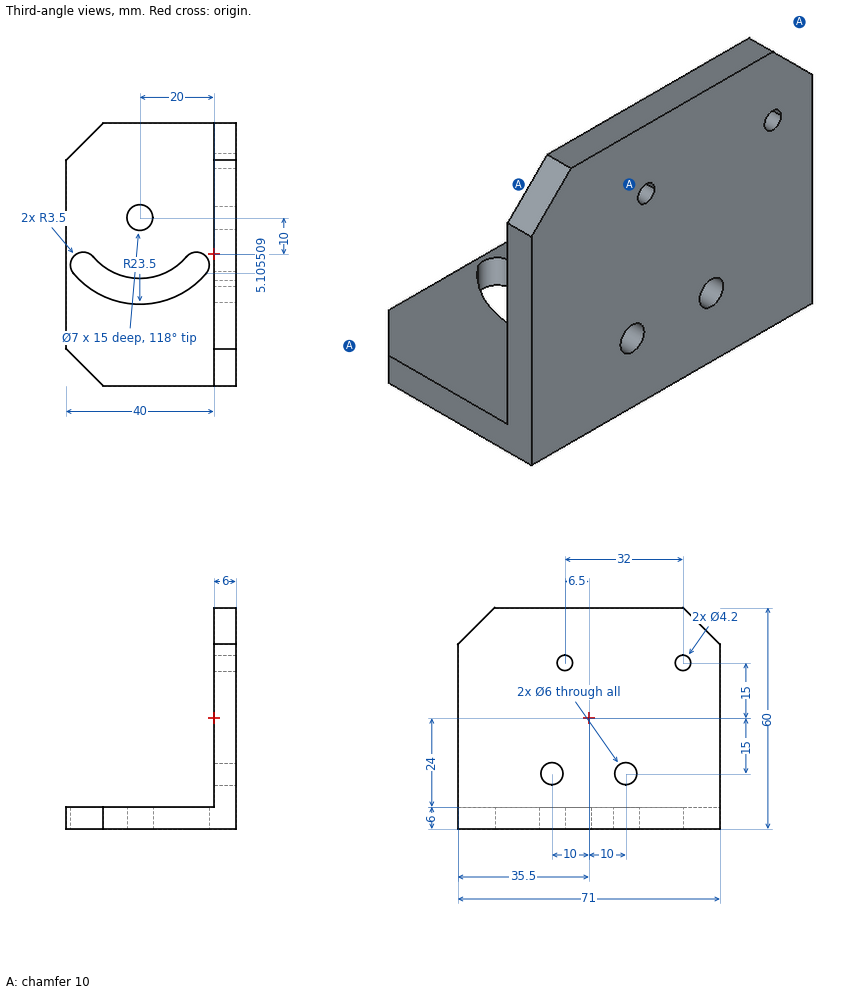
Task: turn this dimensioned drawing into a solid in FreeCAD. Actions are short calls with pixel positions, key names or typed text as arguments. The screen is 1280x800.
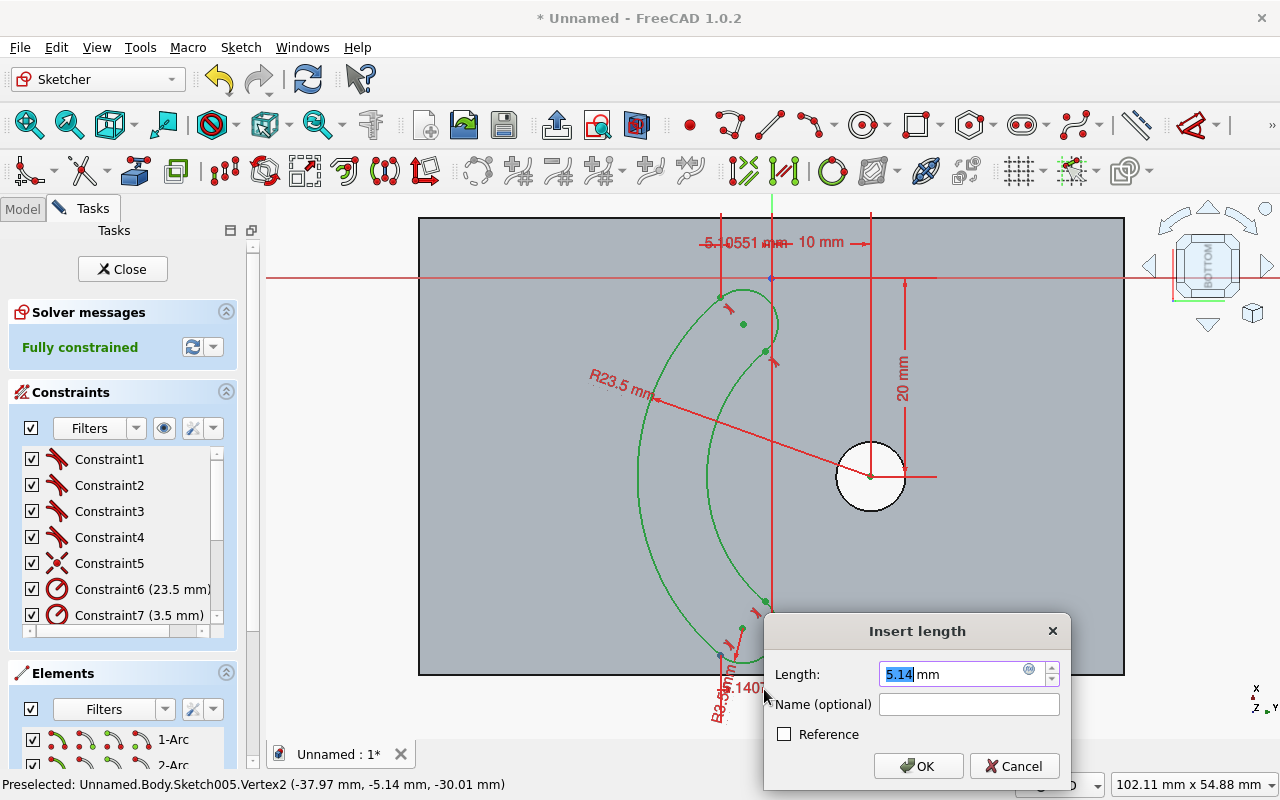
text(5.105509)
key(Return)
key(Escape)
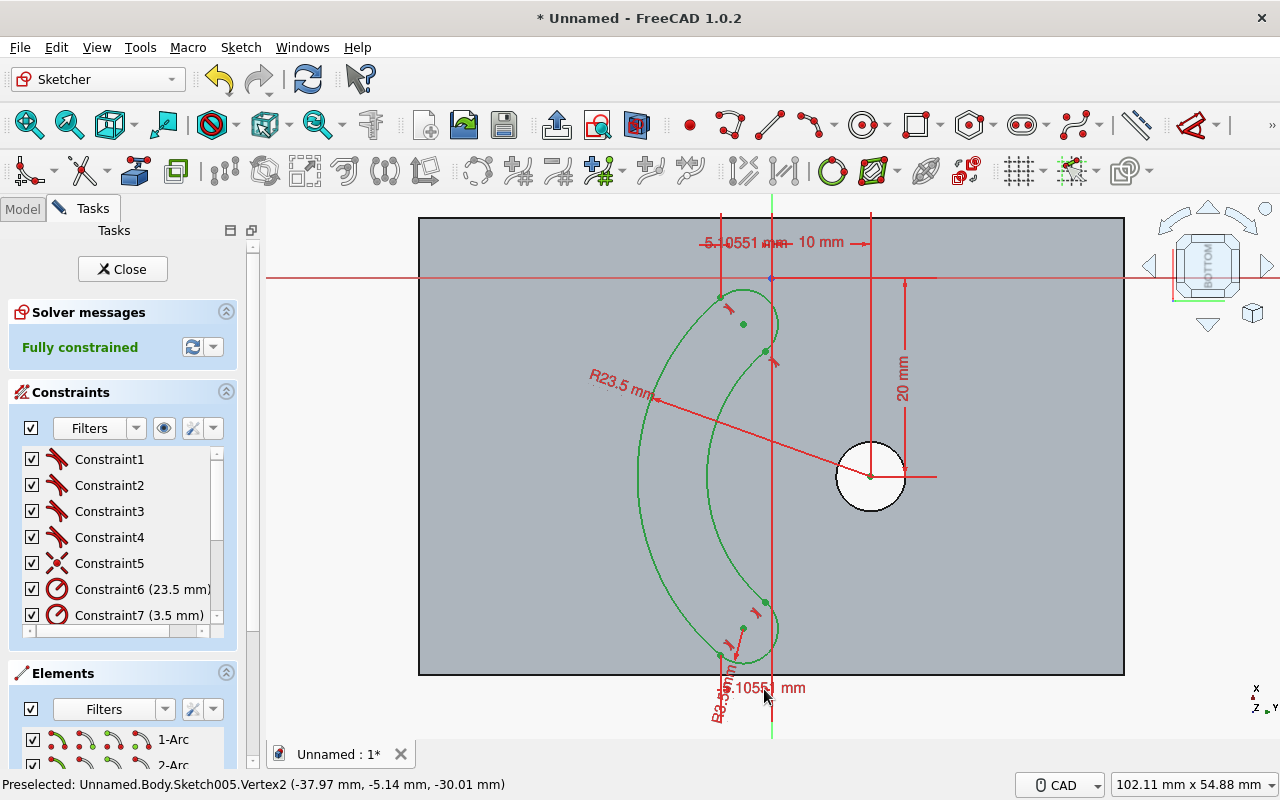
click(123, 269)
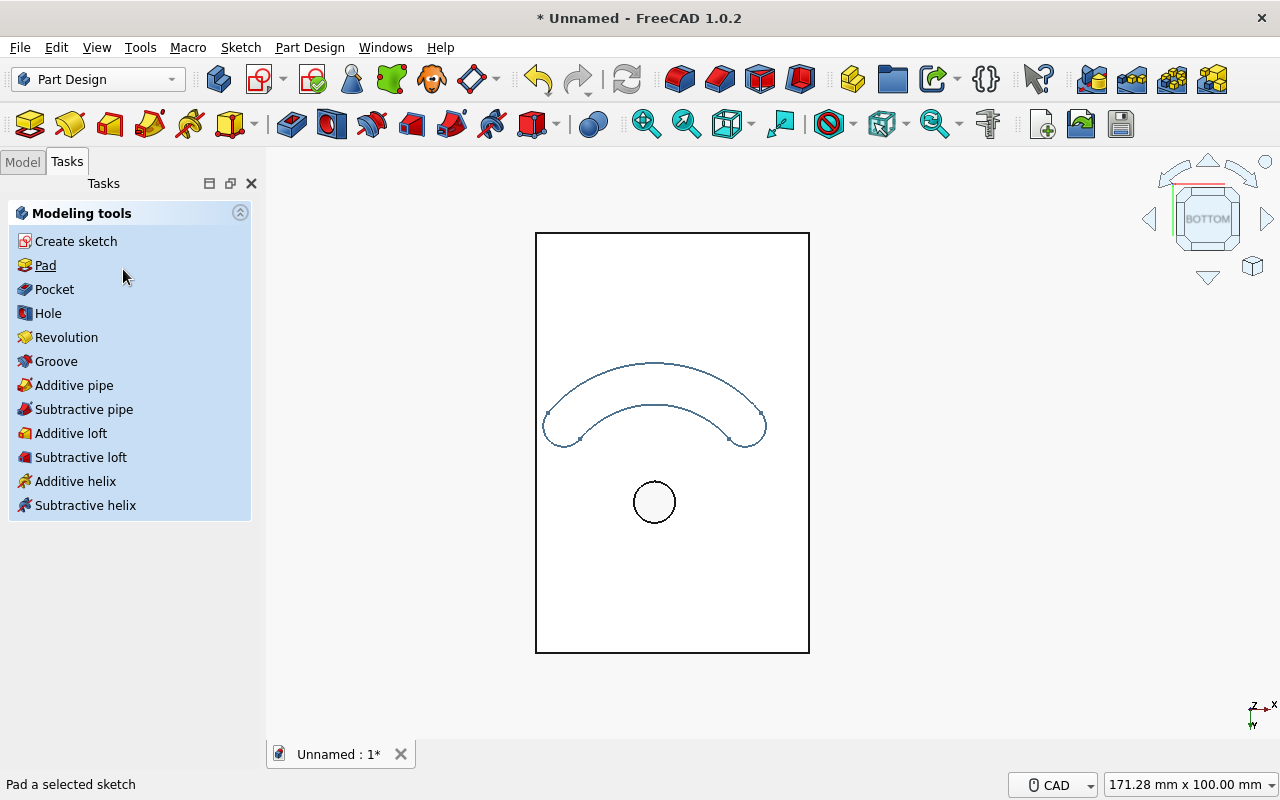
click(292, 124)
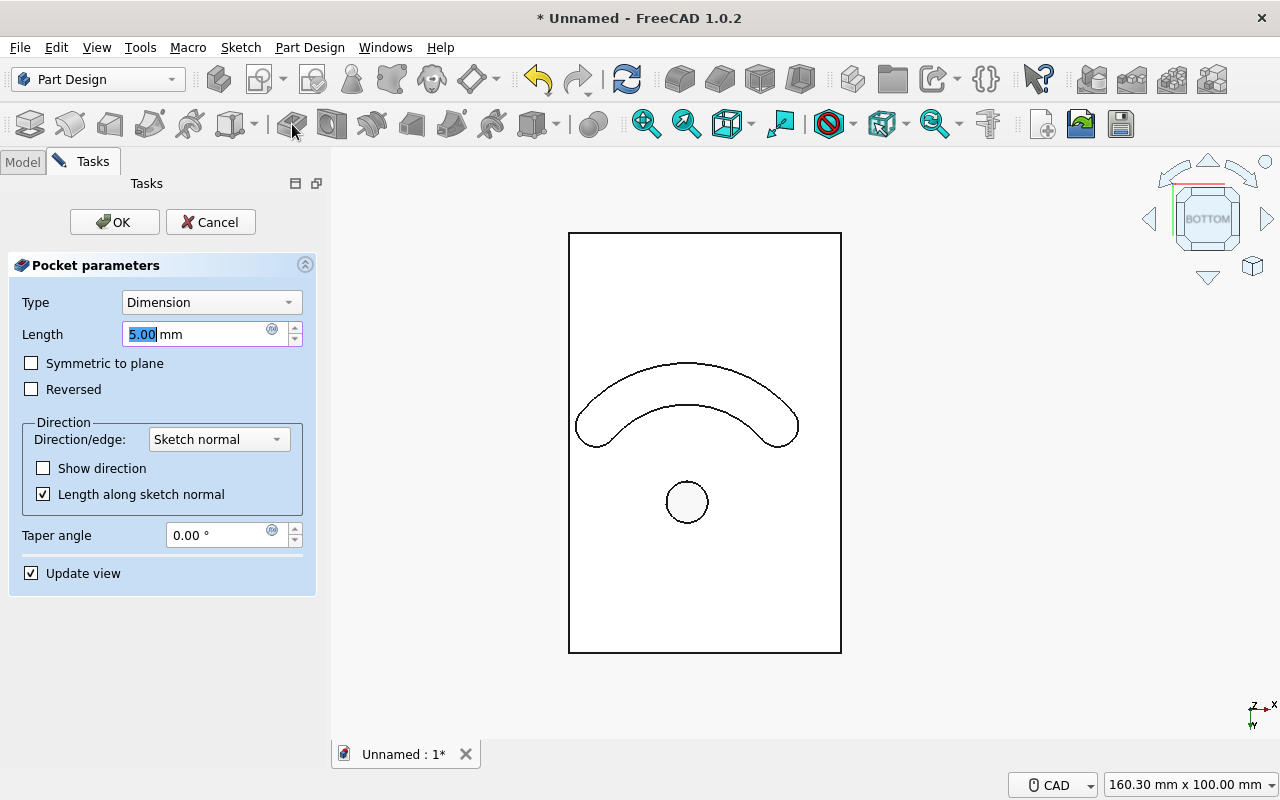
click(212, 302)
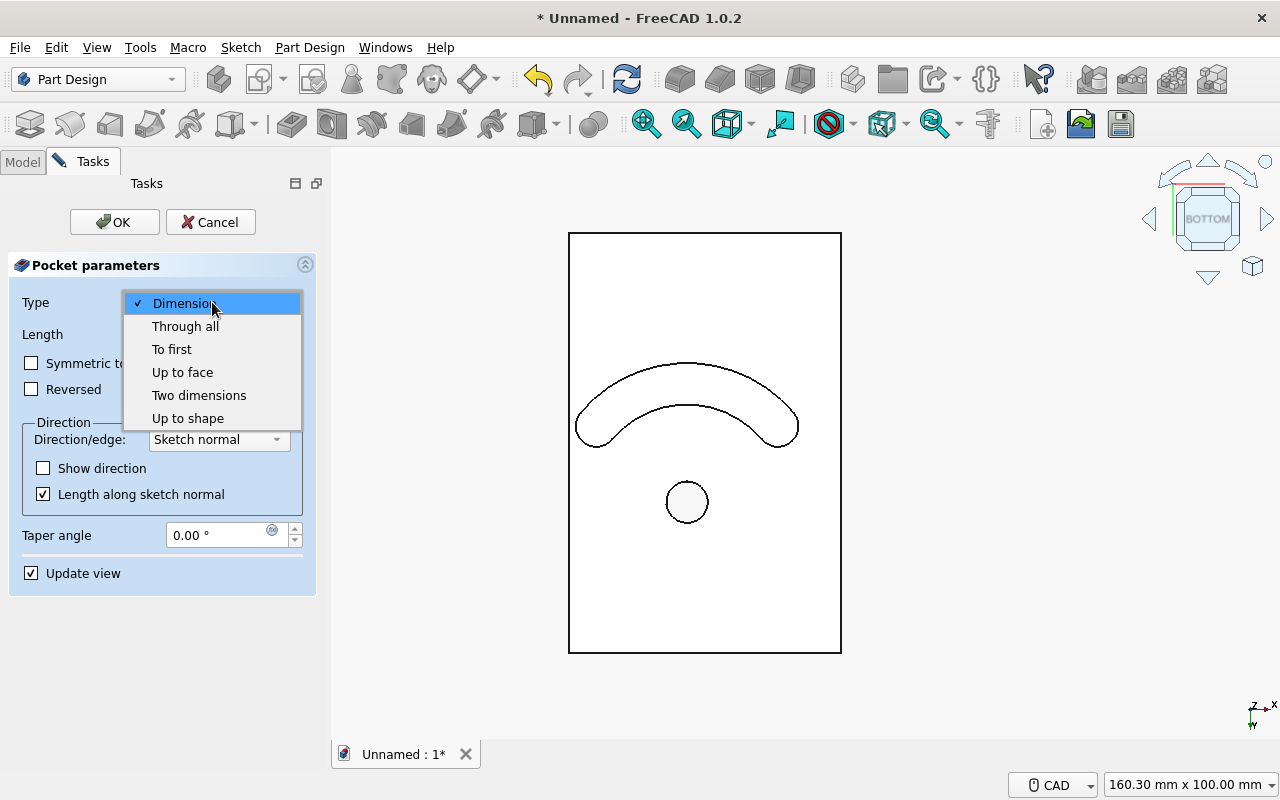
click(212, 326)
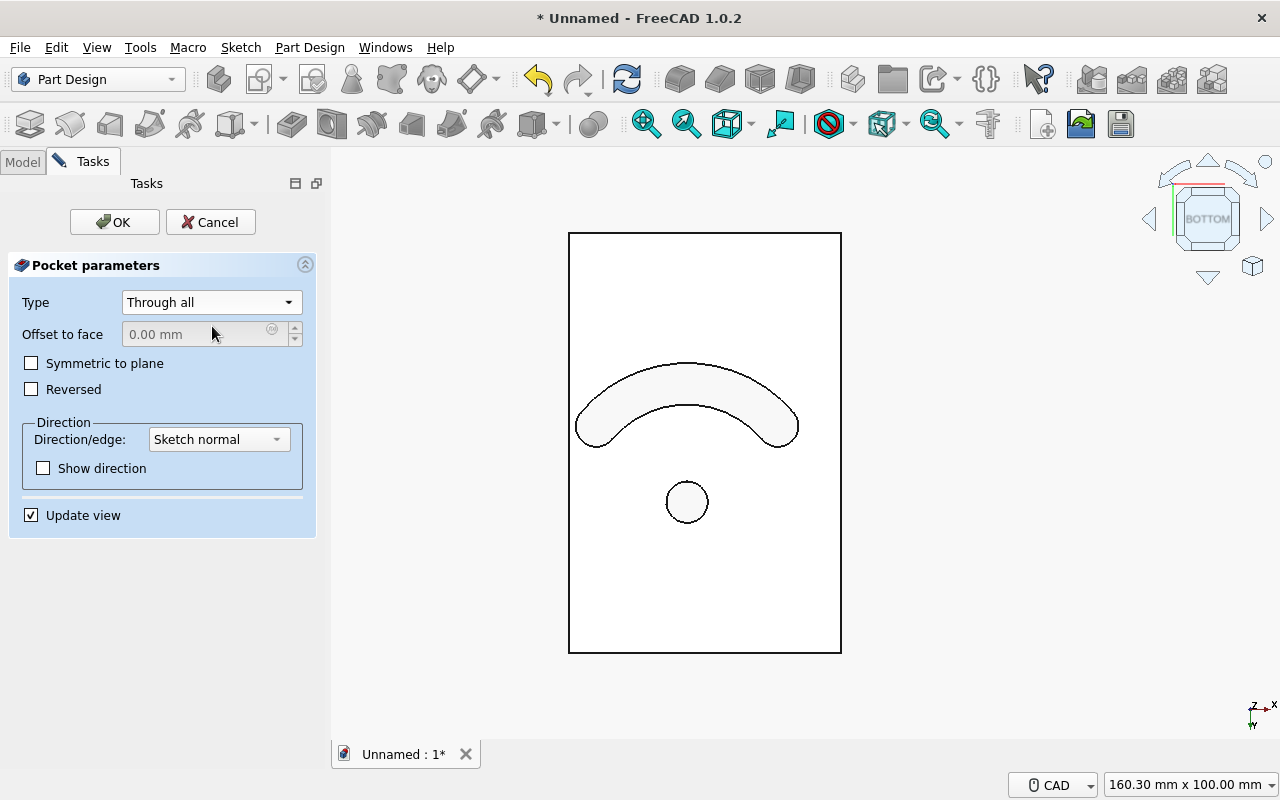
click(115, 222)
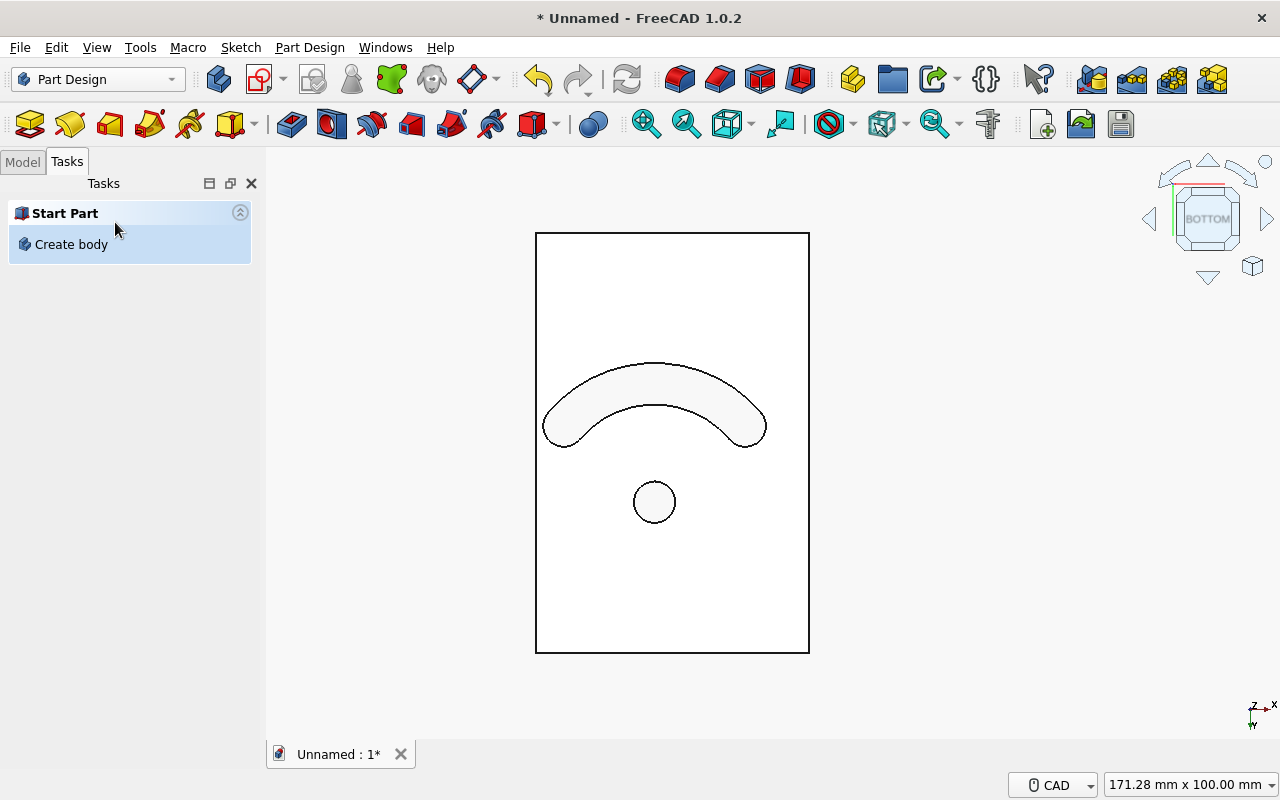
key(0)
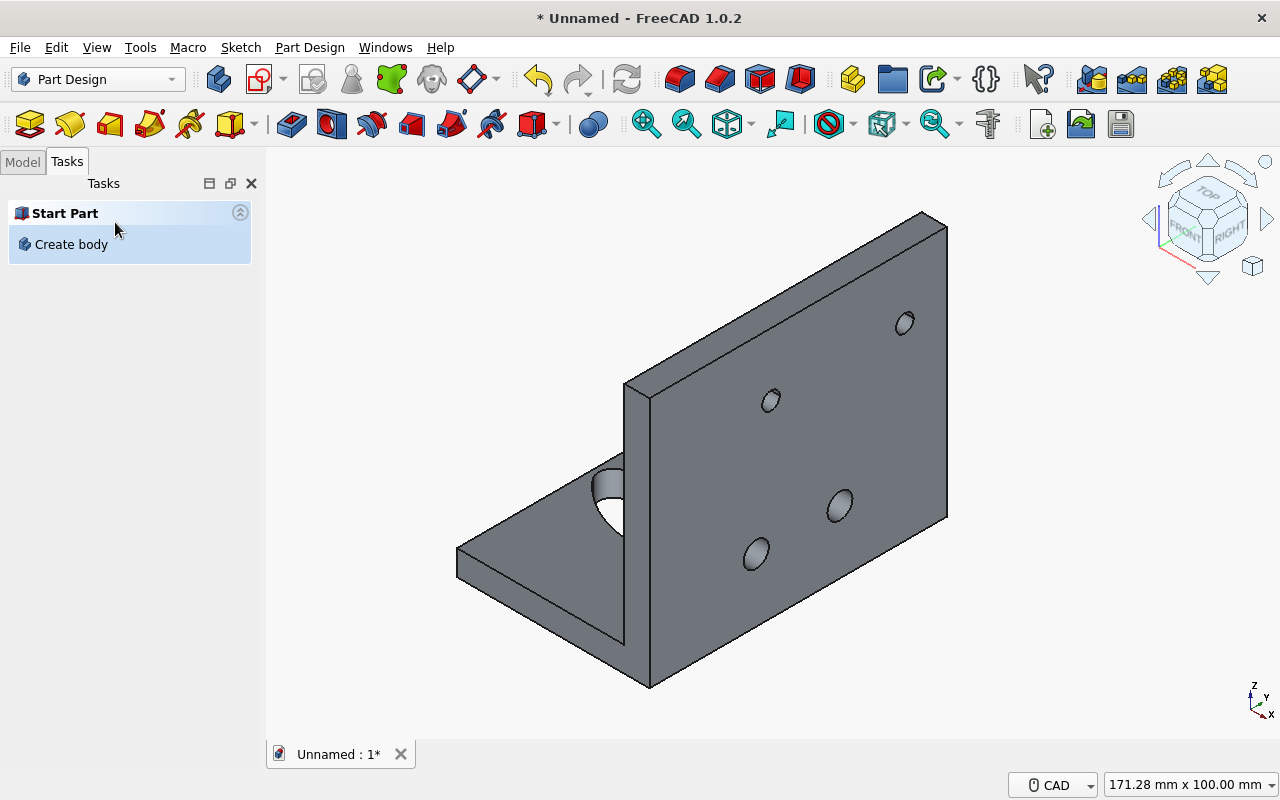
click(648, 124)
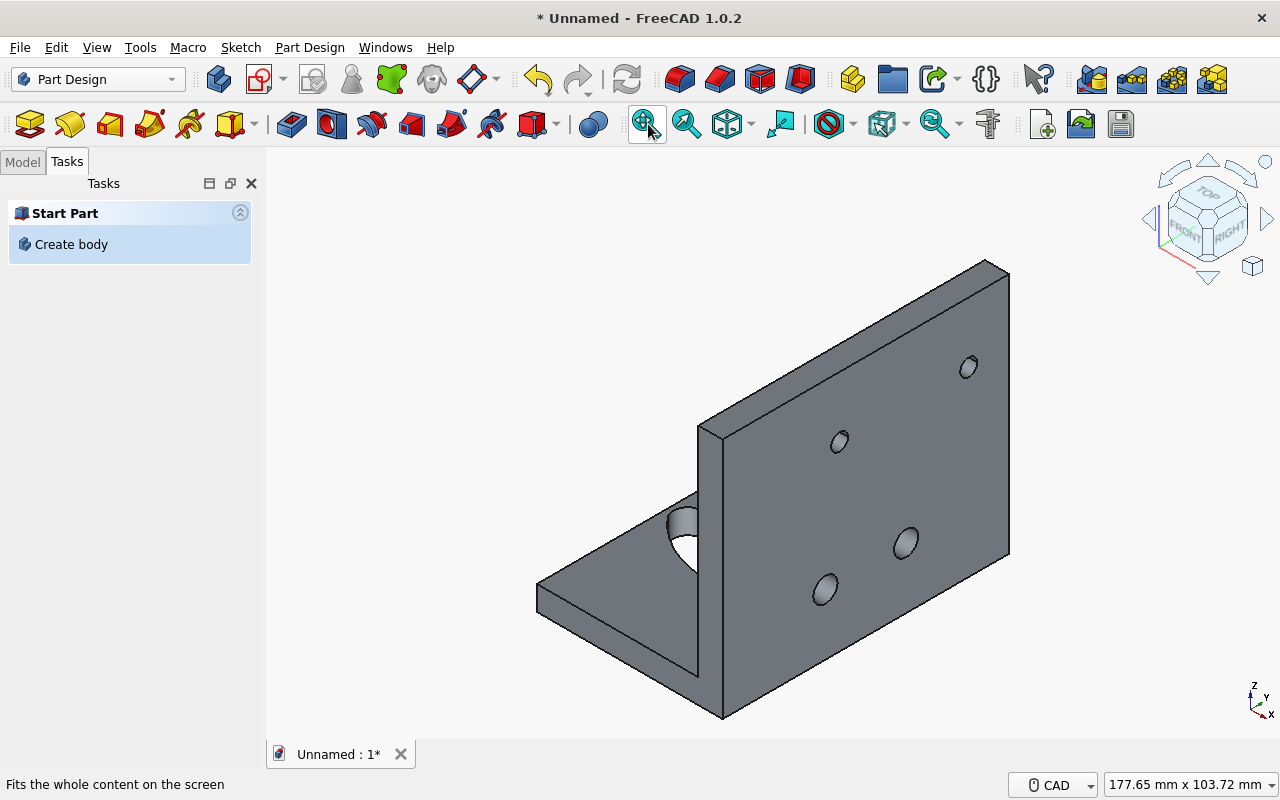
click(710, 432)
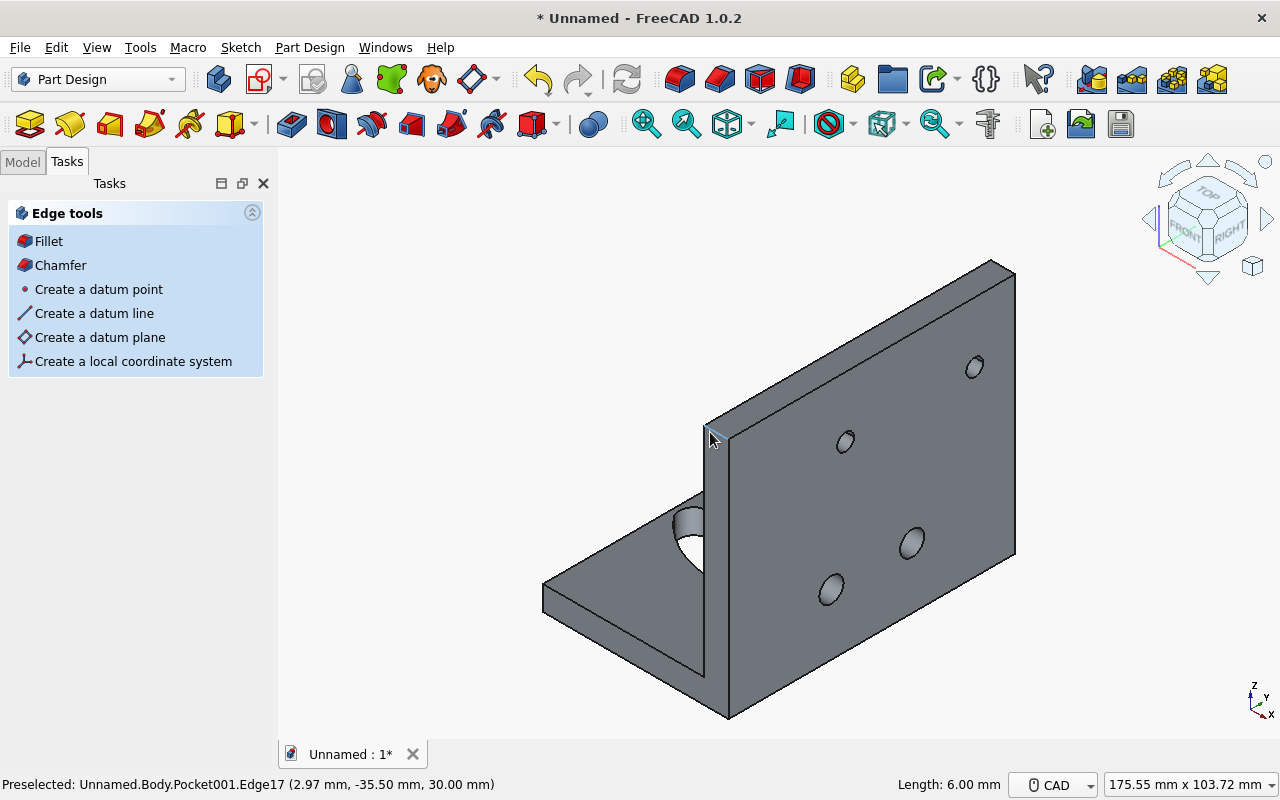
key(2)